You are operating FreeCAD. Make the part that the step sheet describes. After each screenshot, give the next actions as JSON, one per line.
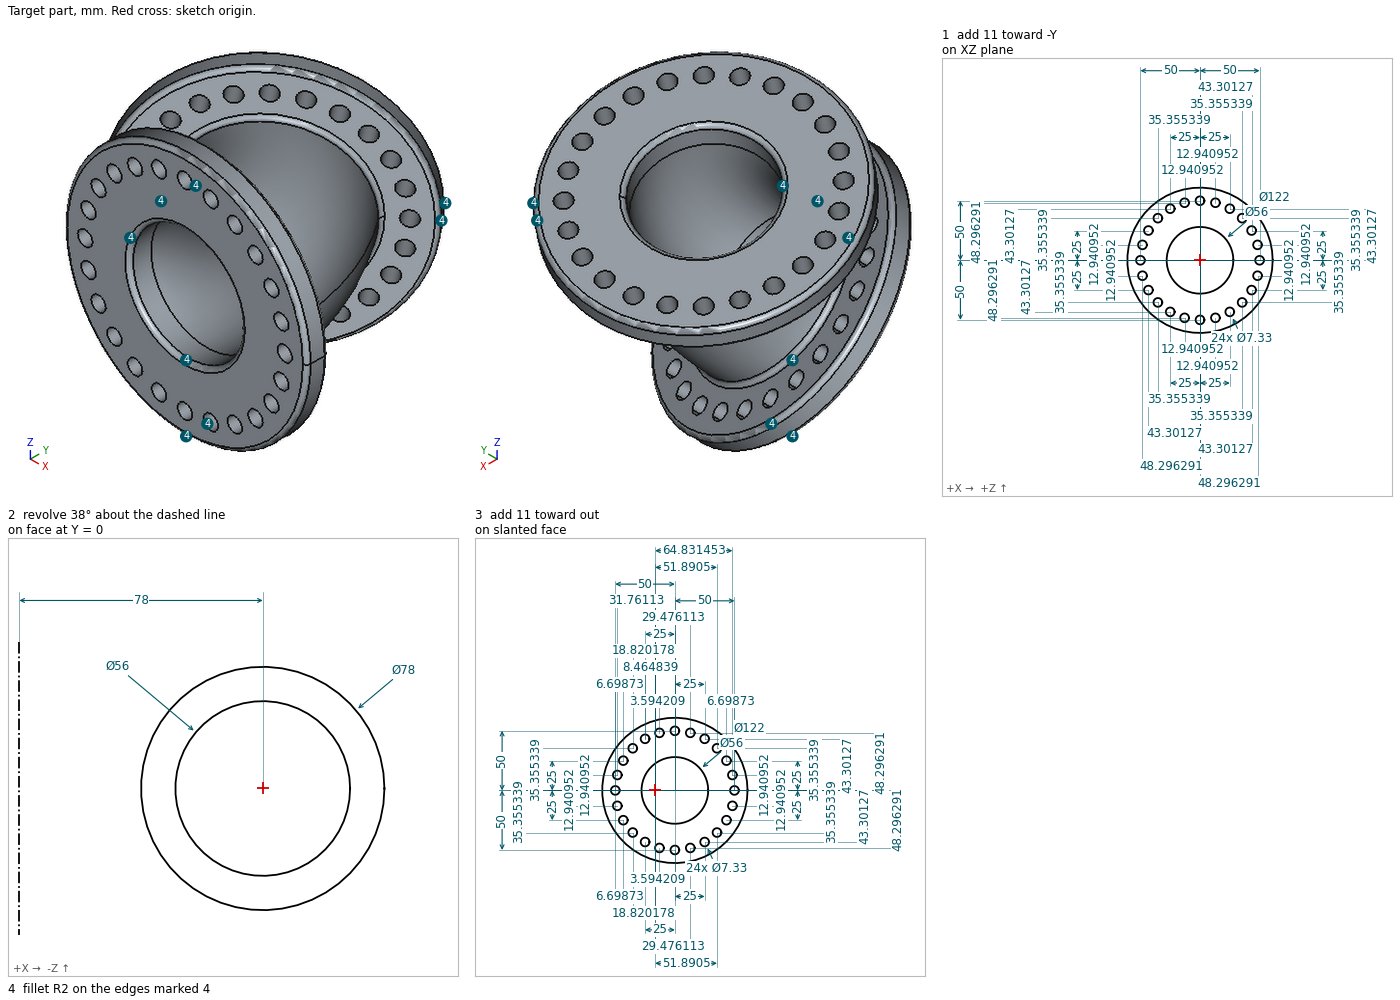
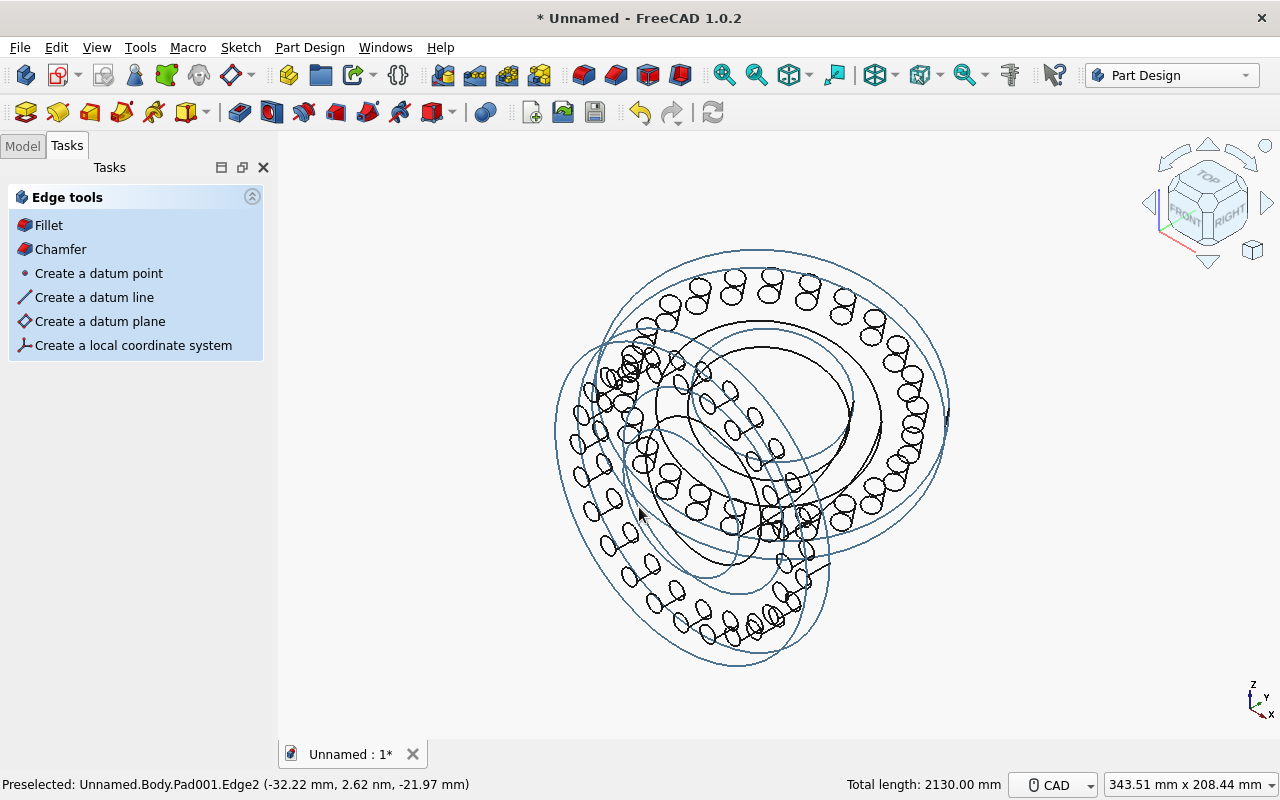
{"action": "left_click", "coordinate": [656, 405], "text": "ctrl"}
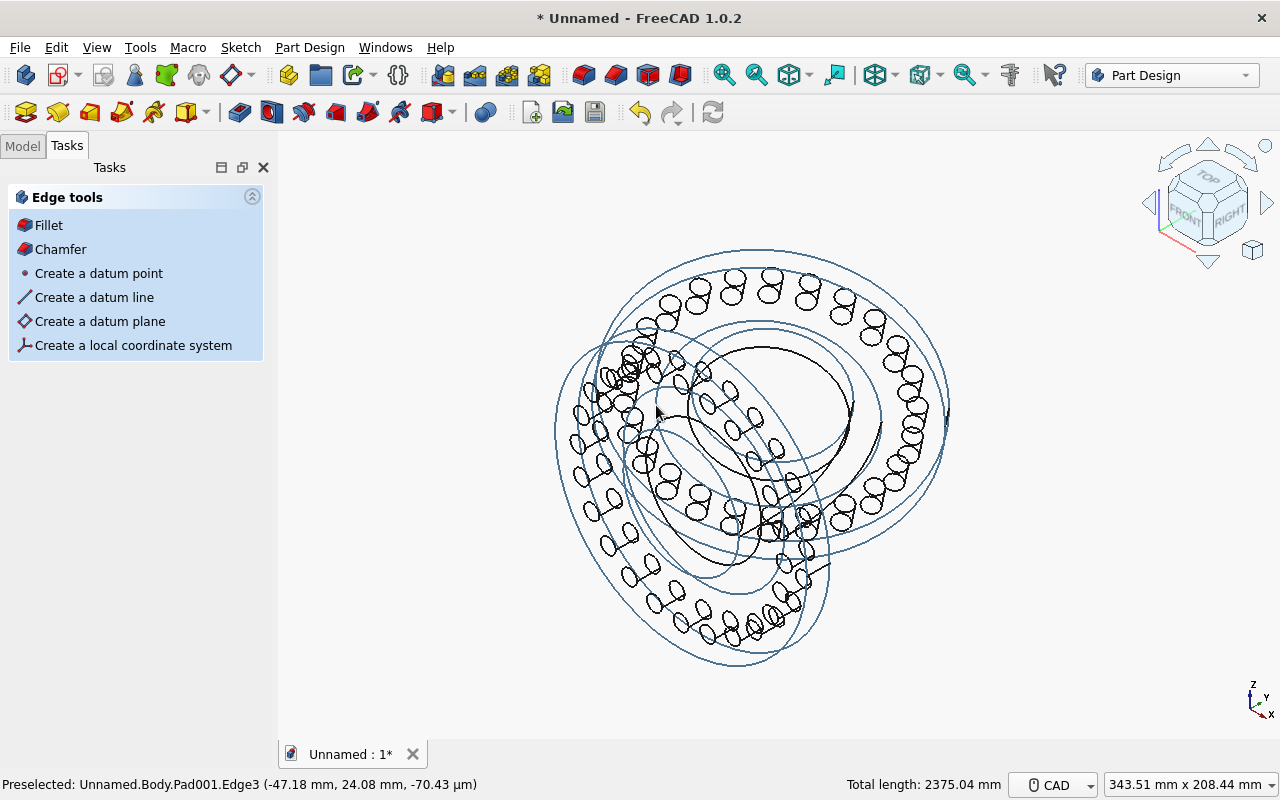
{"action": "key", "text": "v 1"}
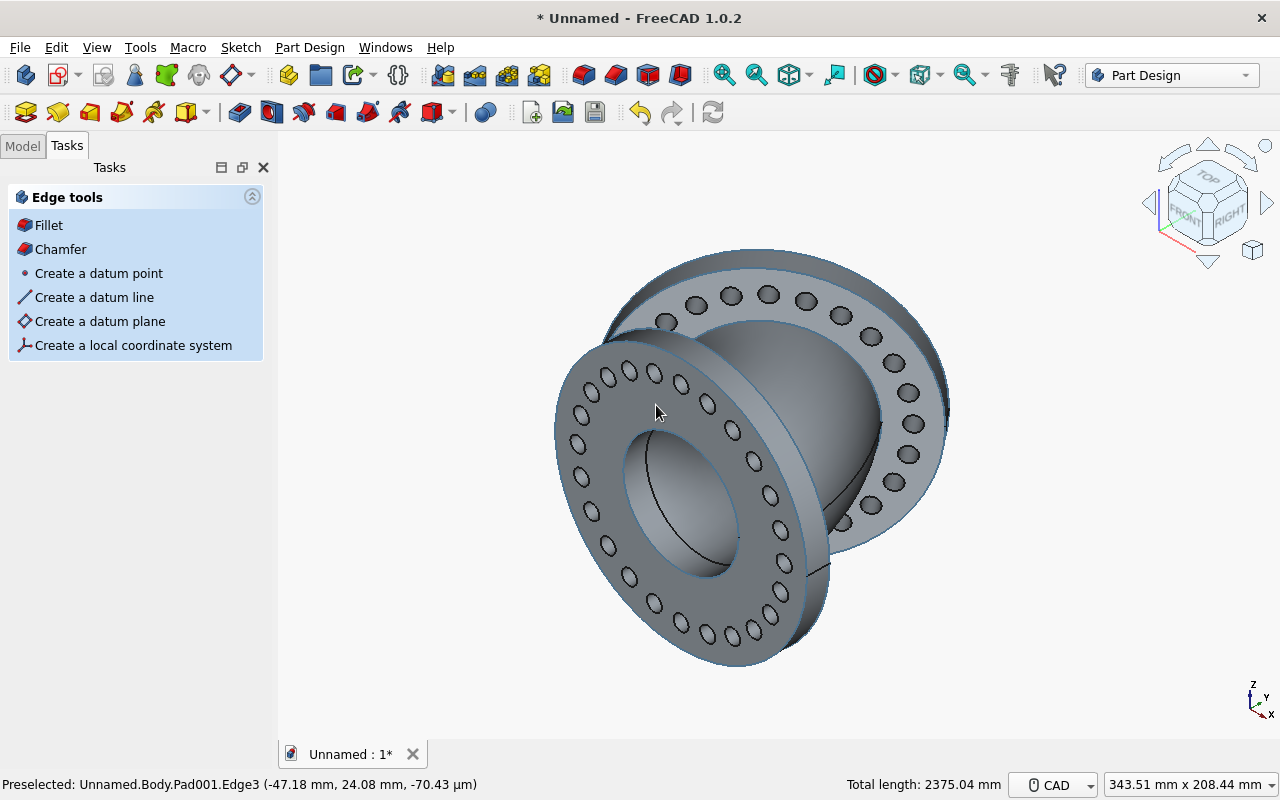
{"action": "left_click", "coordinate": [584, 76]}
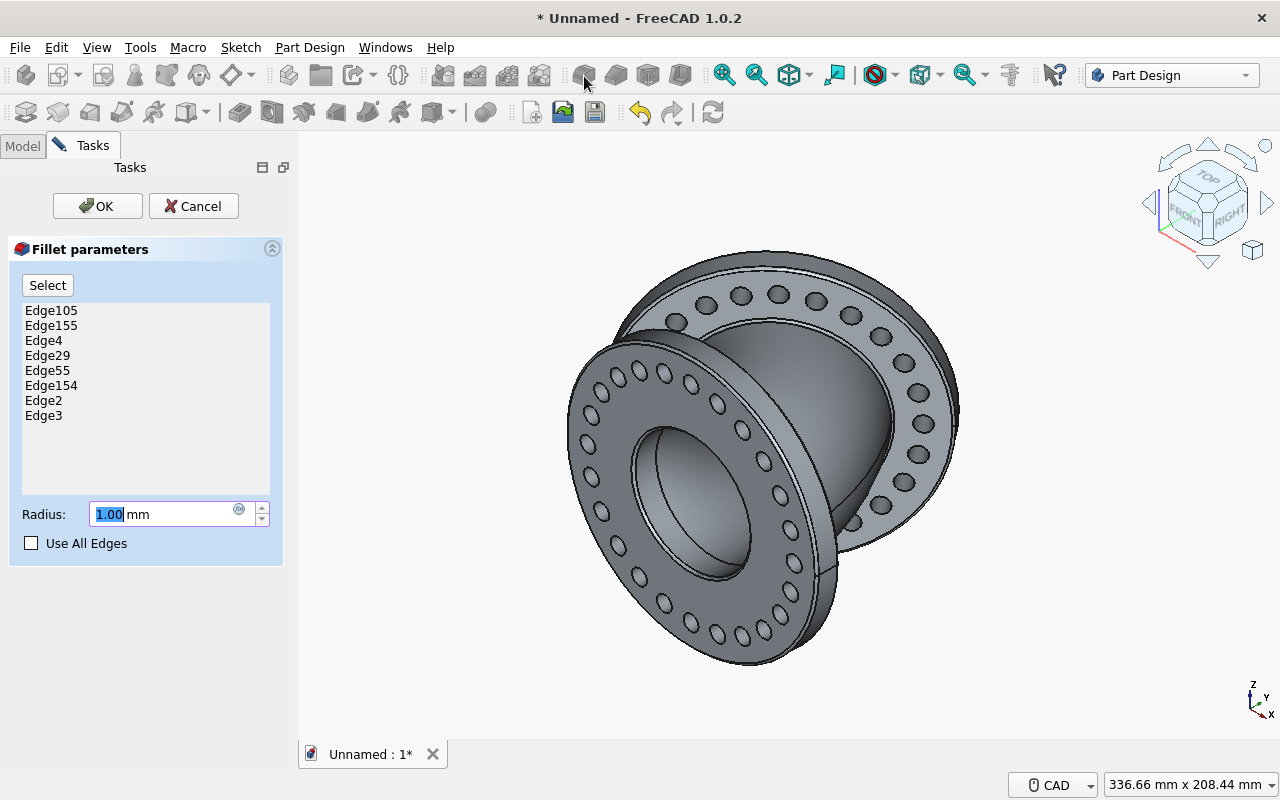
{"action": "type", "text": "2"}
{"action": "key", "text": "Tab"}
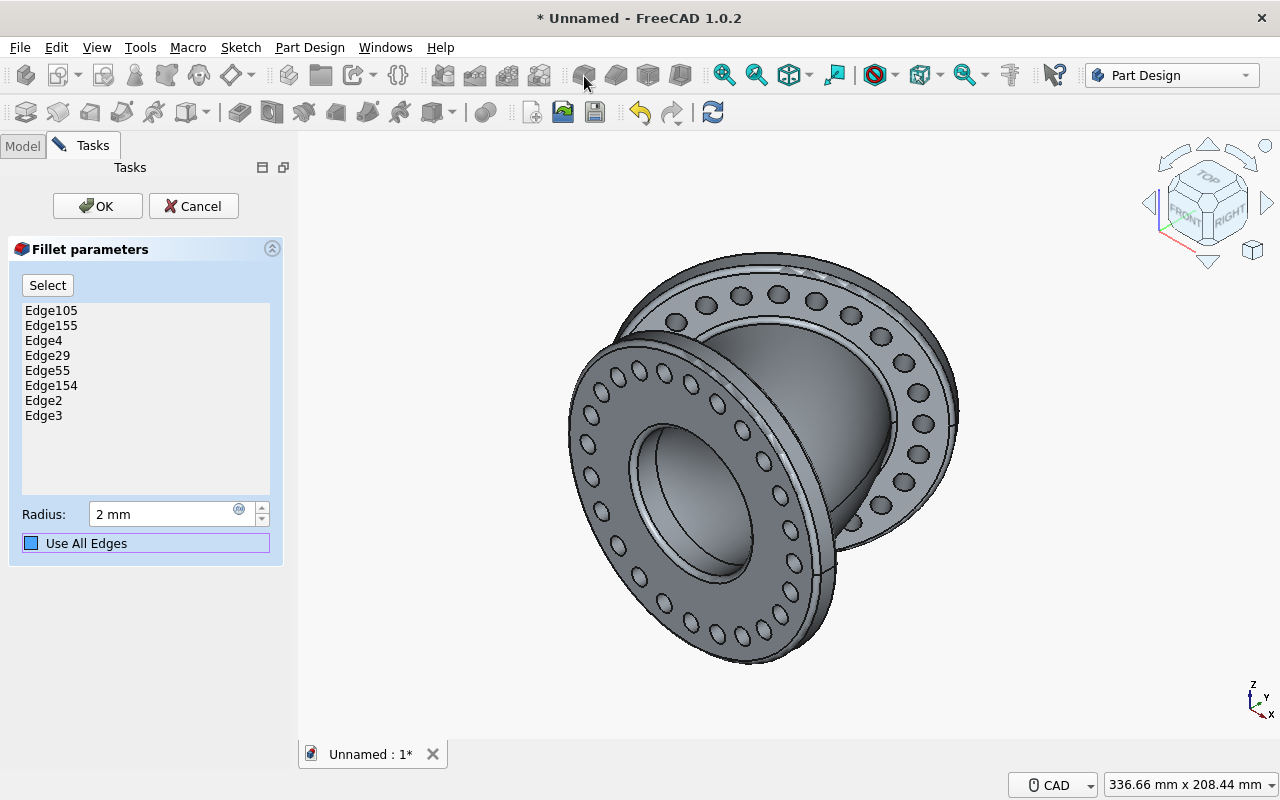
{"action": "left_click", "coordinate": [98, 206]}